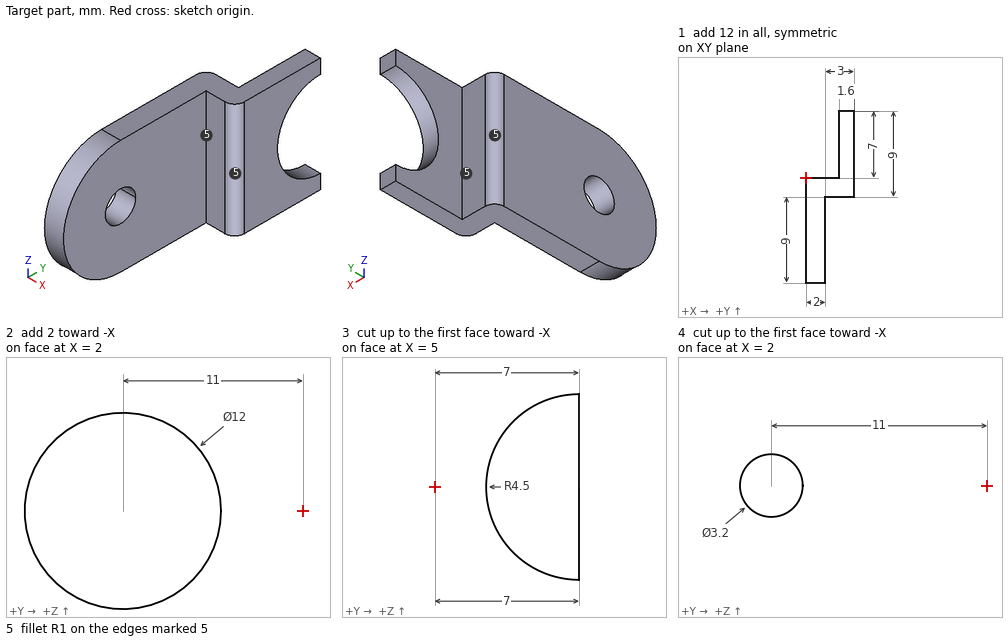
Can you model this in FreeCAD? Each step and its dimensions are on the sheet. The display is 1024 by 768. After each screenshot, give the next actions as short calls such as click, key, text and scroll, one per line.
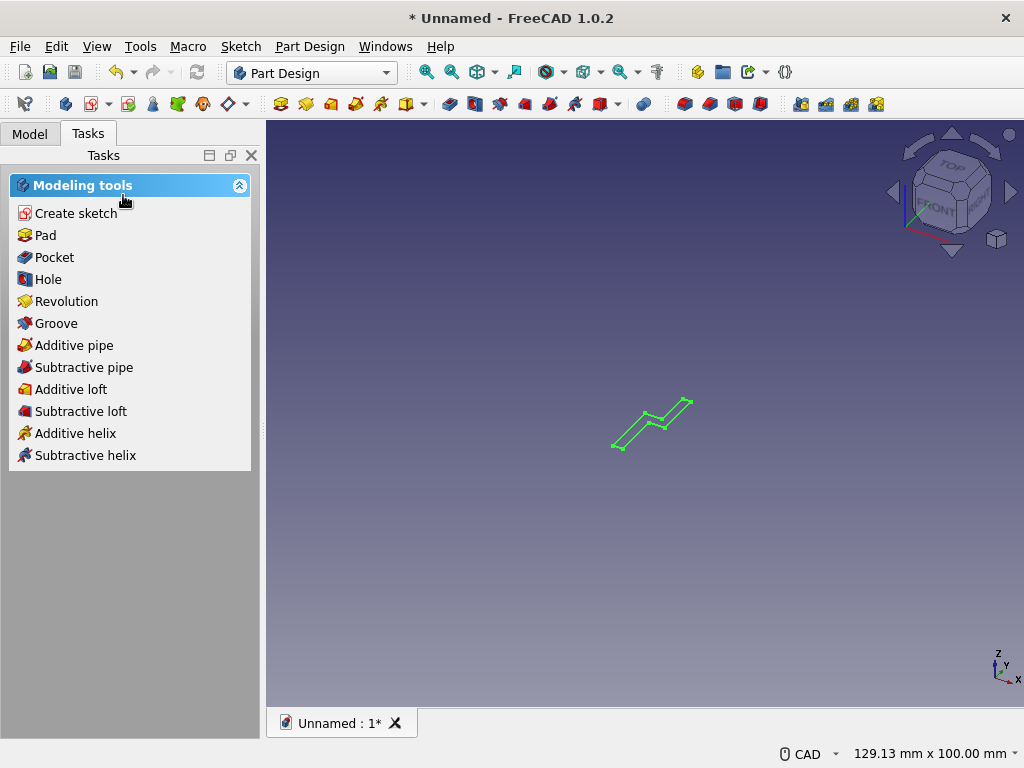
click(281, 104)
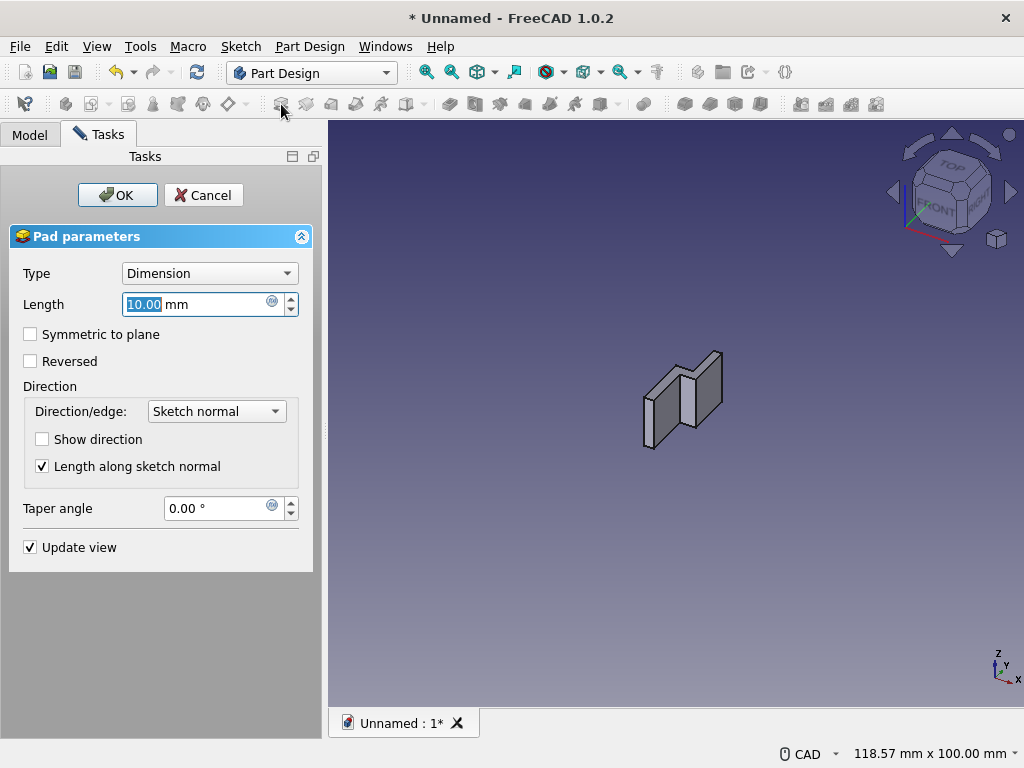
text(12)
key(Tab)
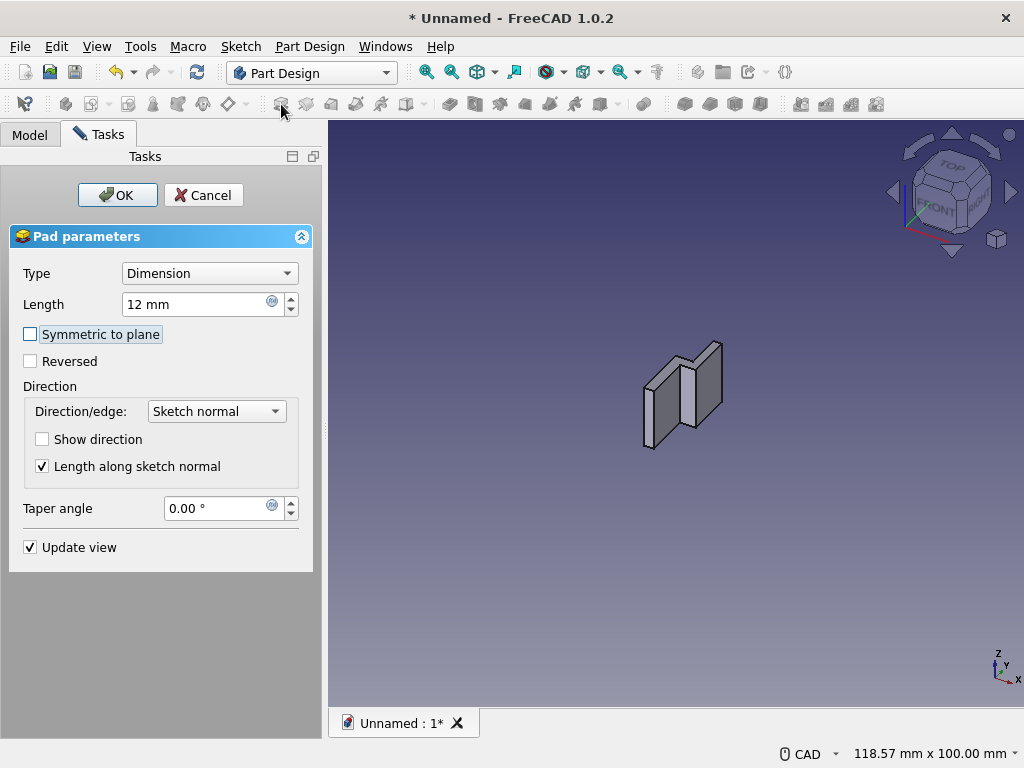
click(31, 334)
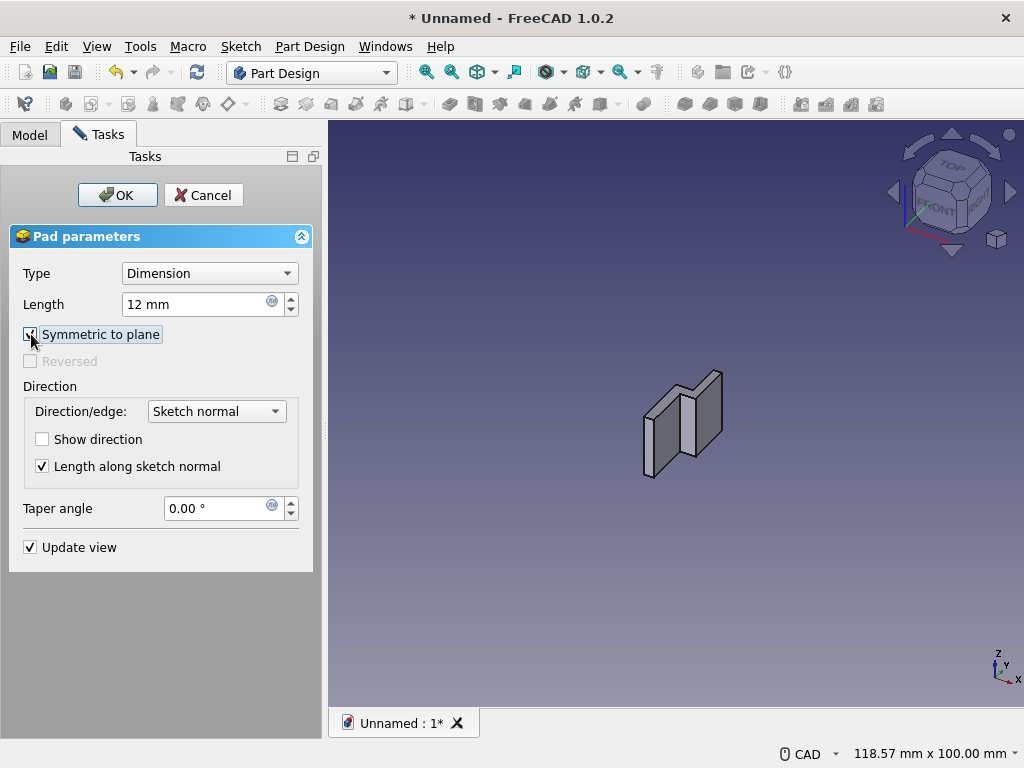
click(118, 195)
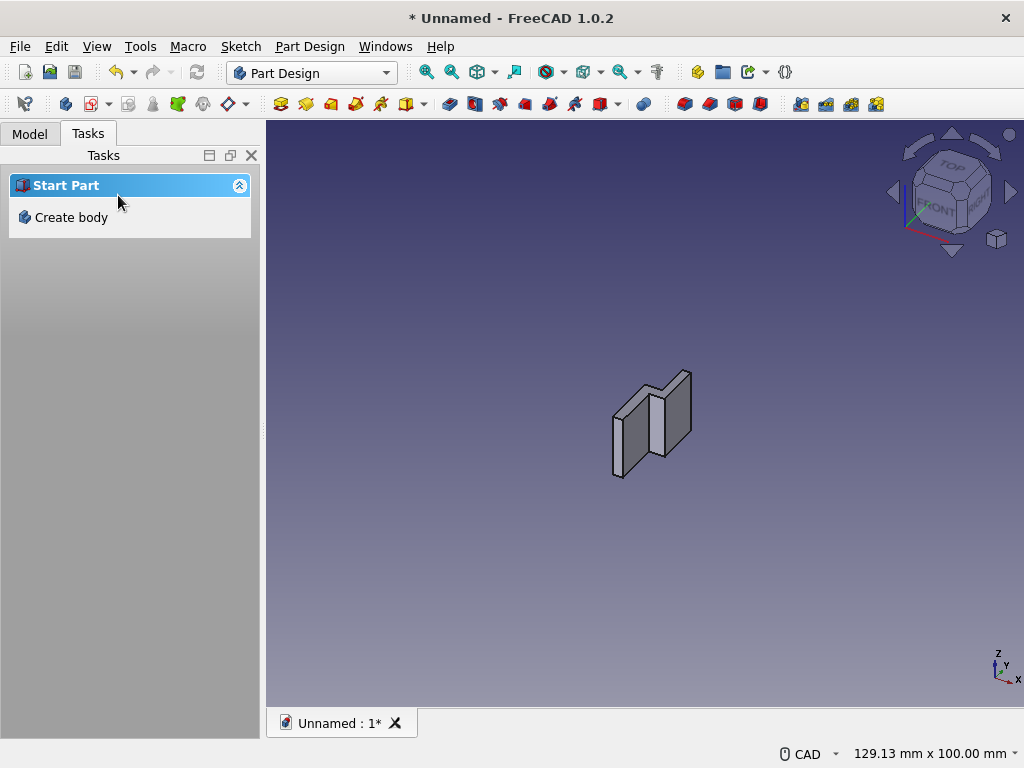
key(v)
key(f)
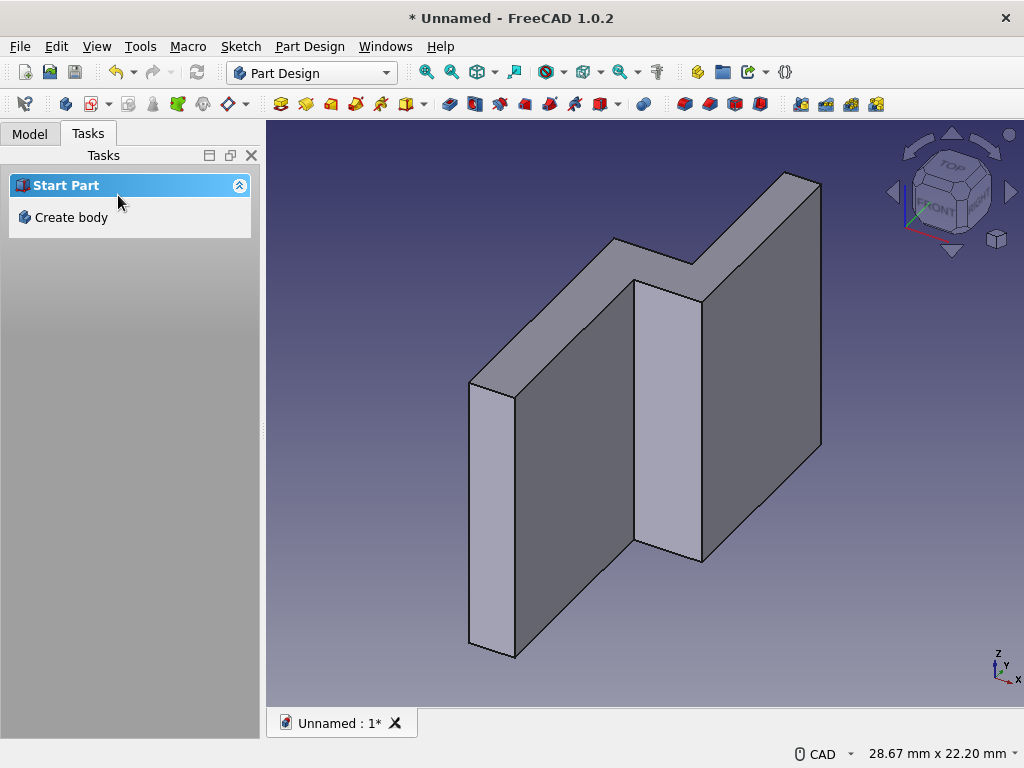
click(574, 468)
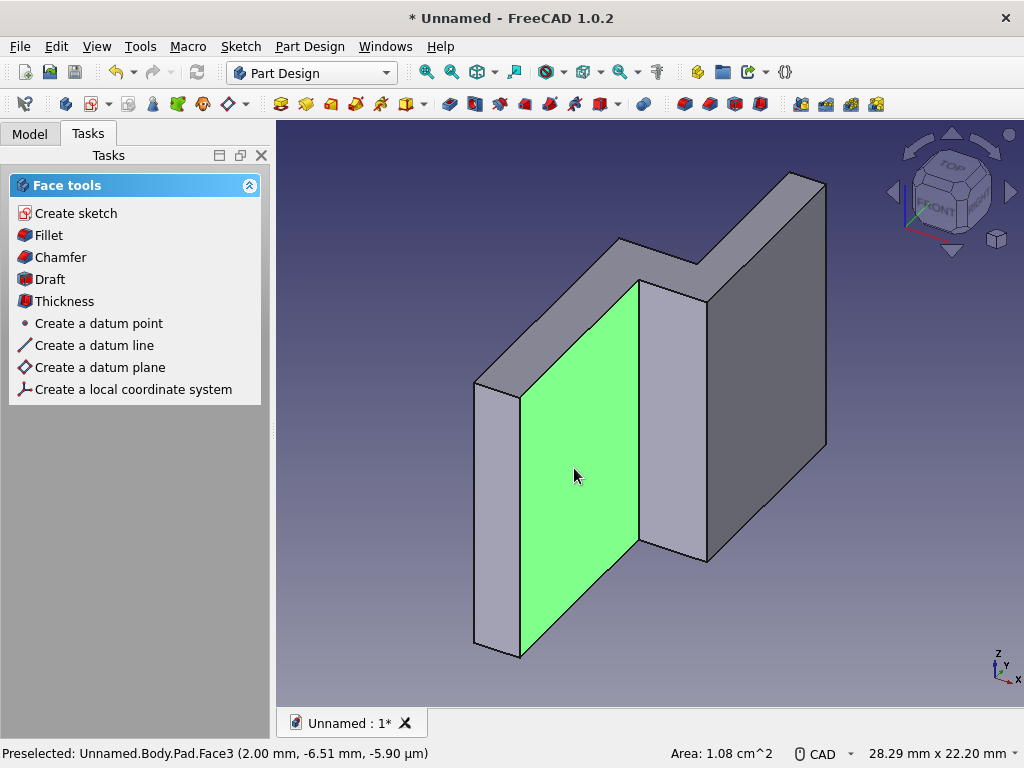
click(90, 104)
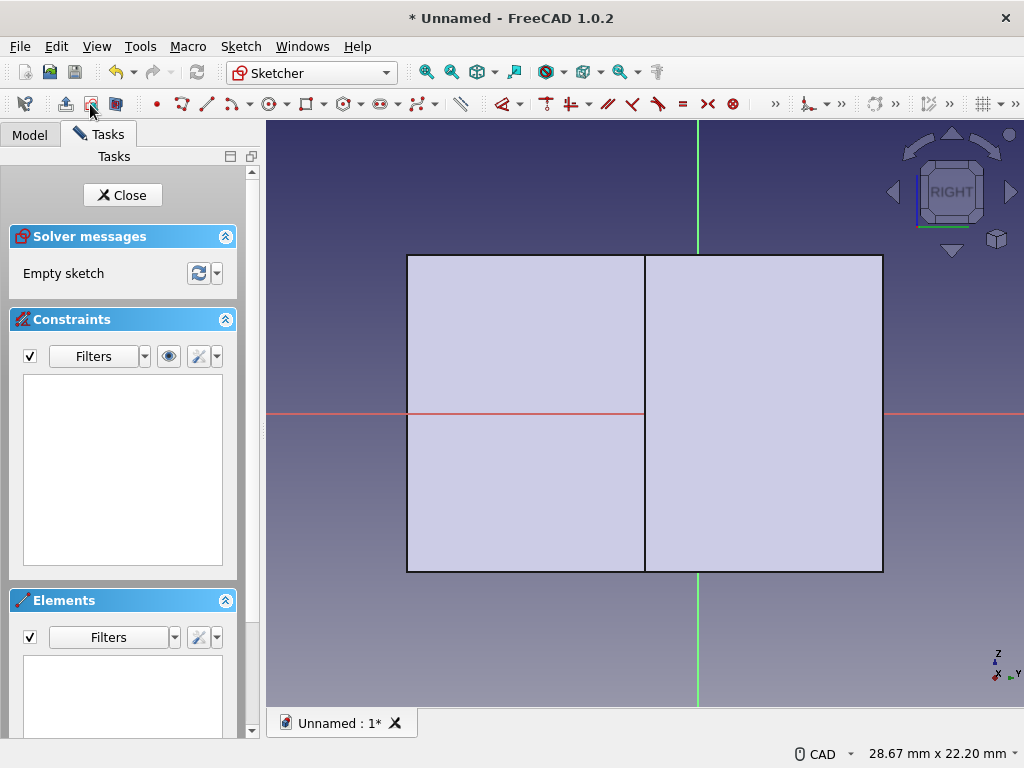
key(q)
key(s)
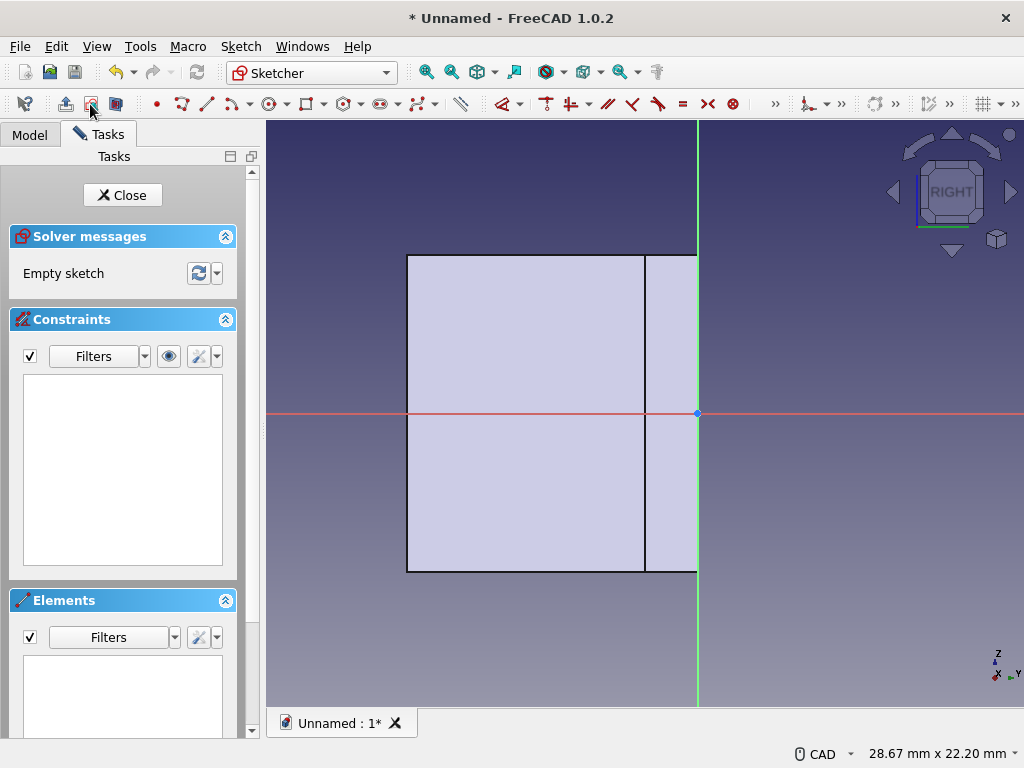
scroll(859, 413, down, 1)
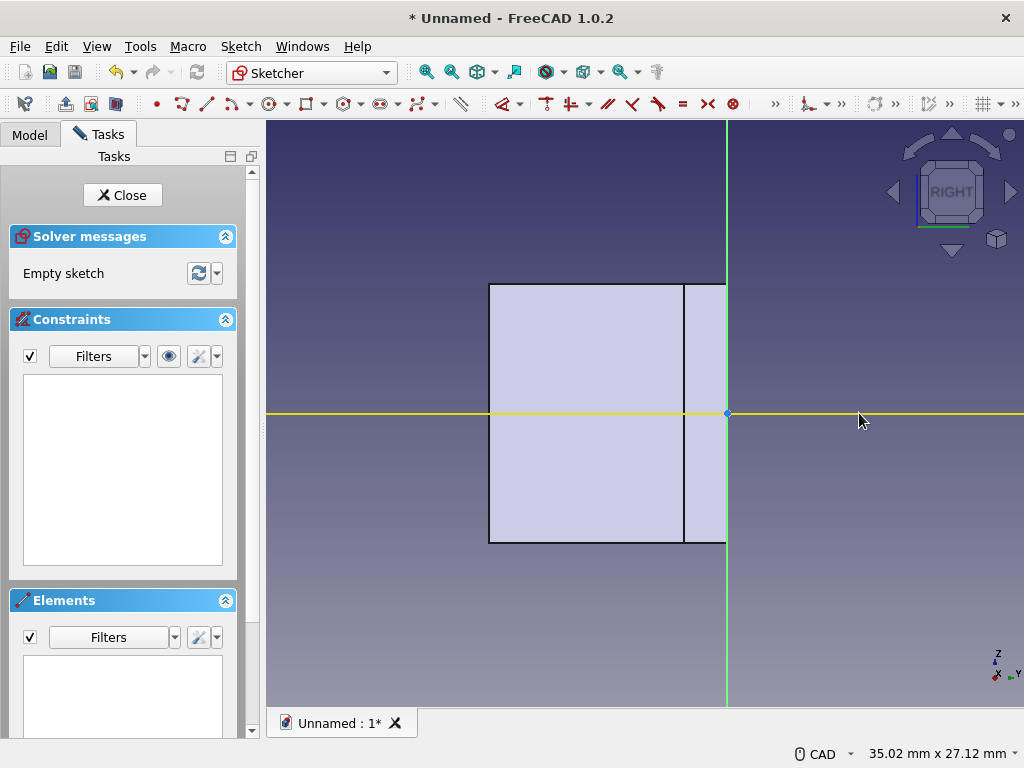
key(g)
key(c)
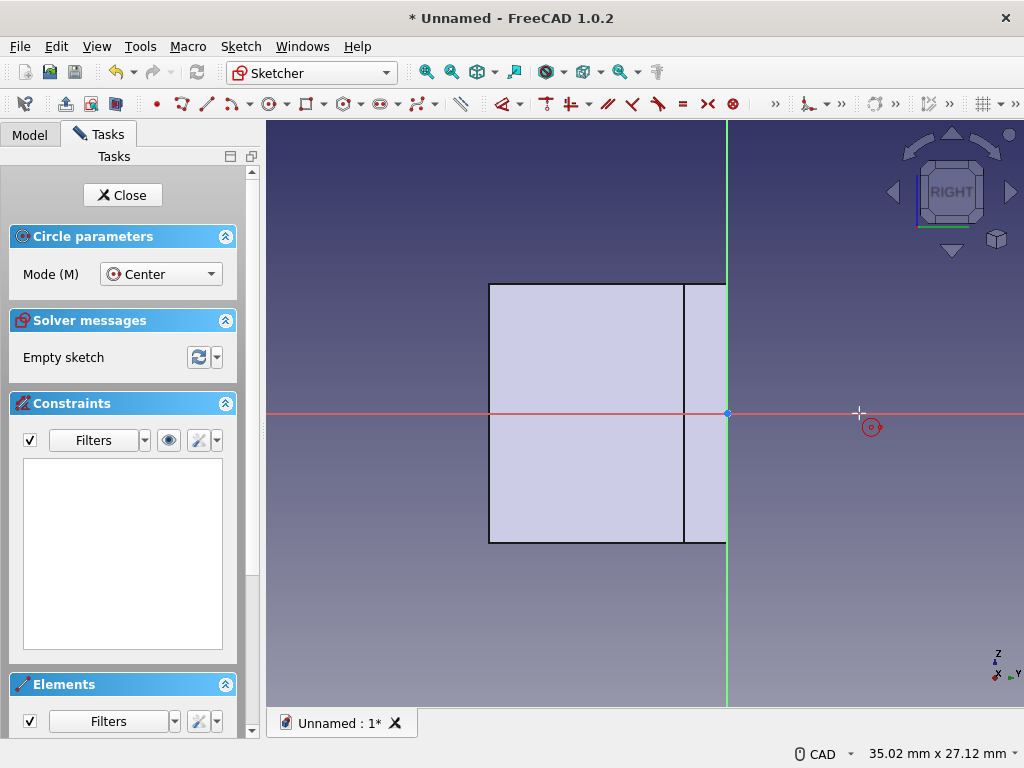
click(489, 414)
move(581, 322)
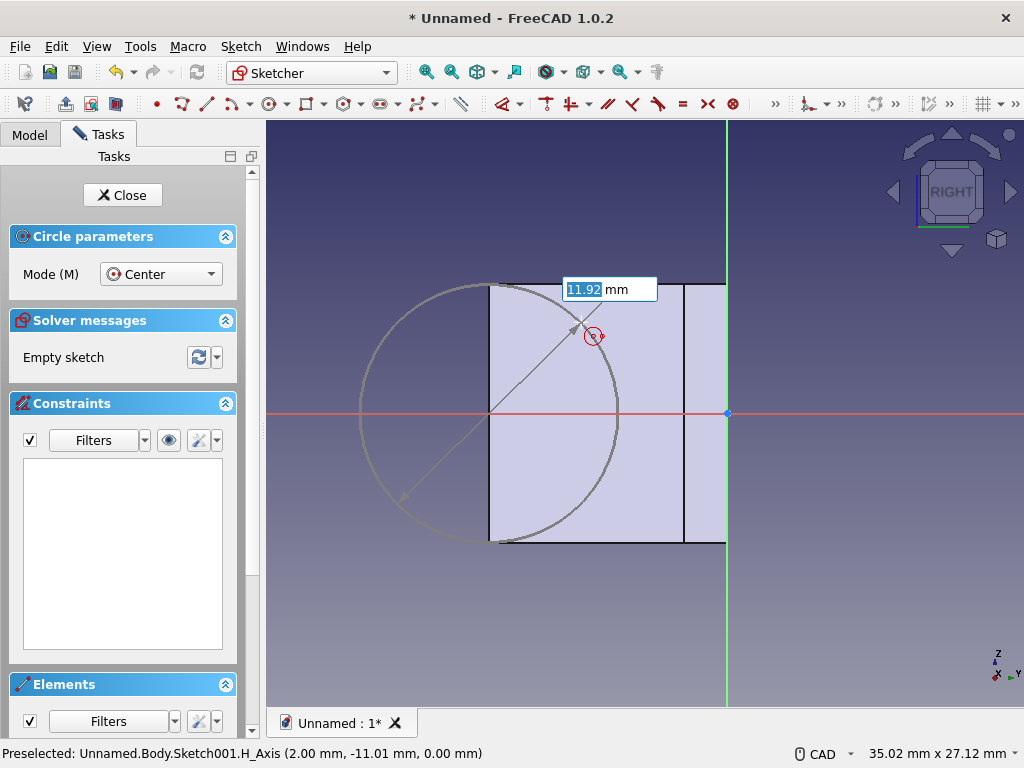
text(12)
key(Return)
key(Escape)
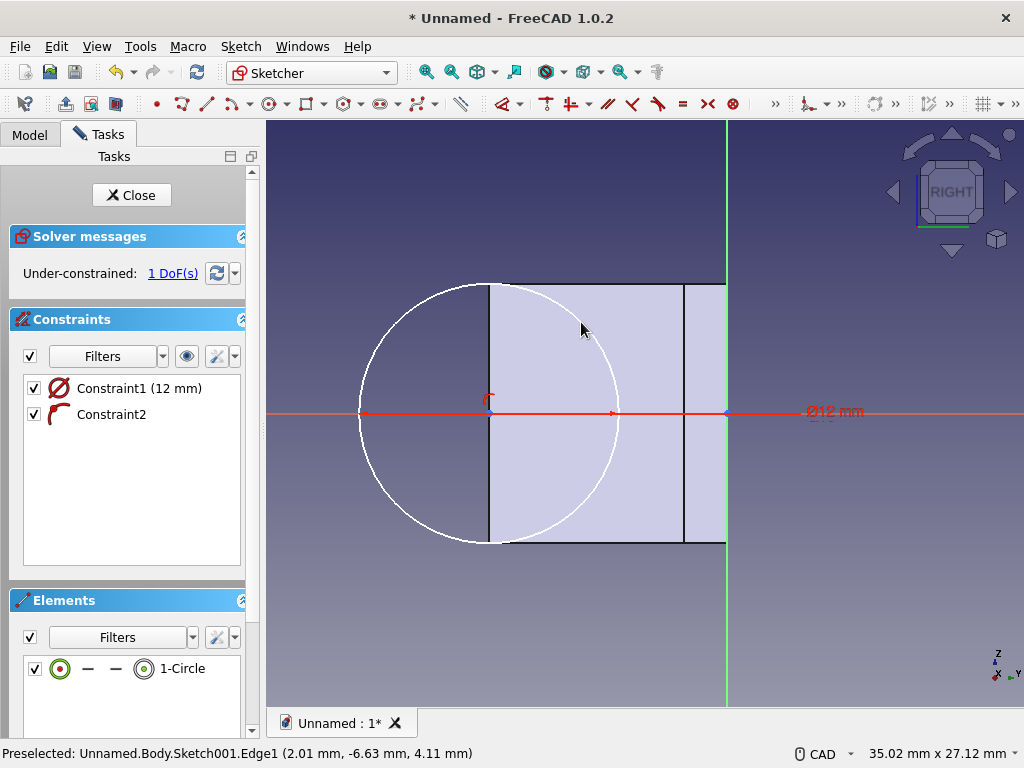
click(502, 104)